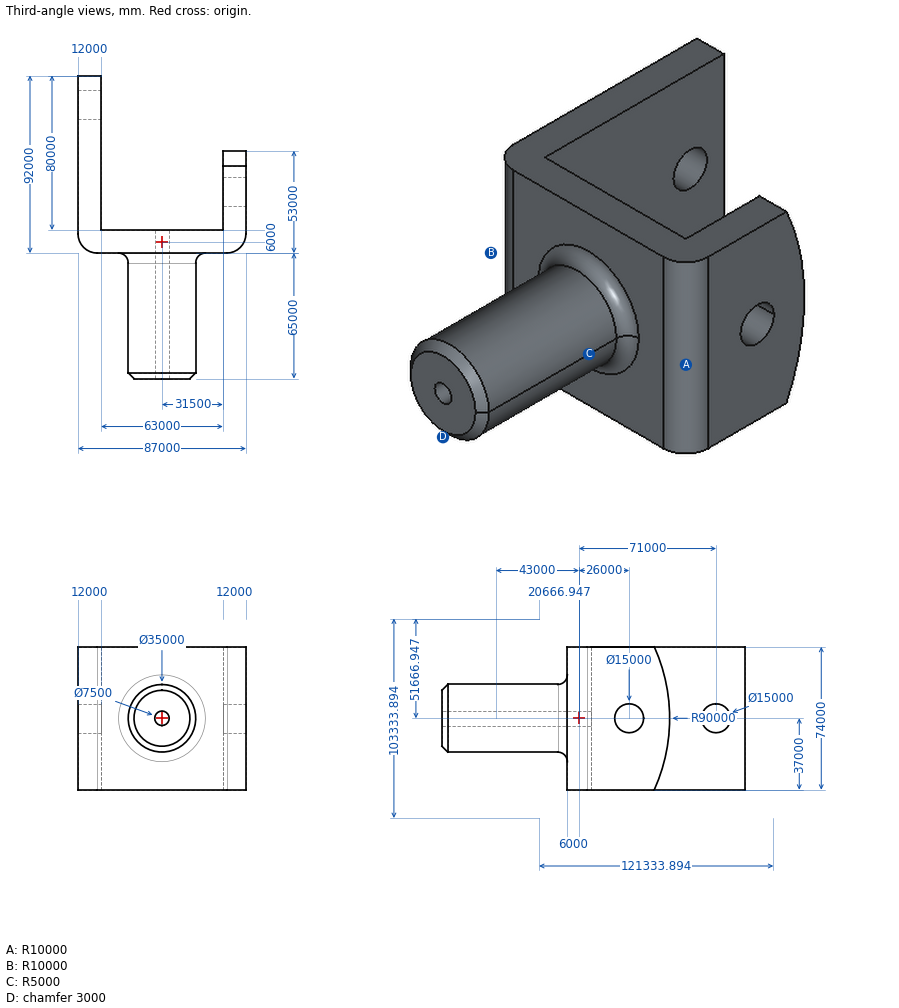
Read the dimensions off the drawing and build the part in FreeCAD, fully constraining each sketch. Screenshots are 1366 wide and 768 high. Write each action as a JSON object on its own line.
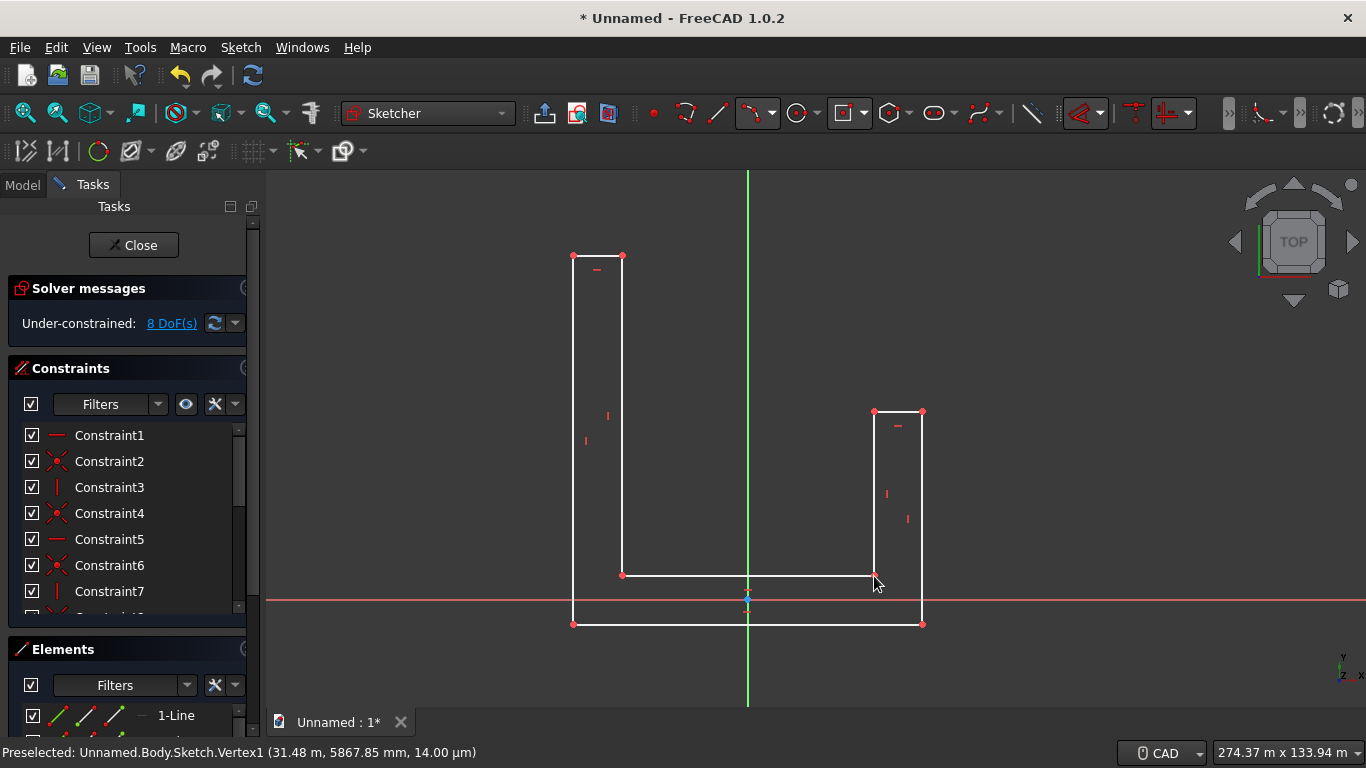
{"action": "left_click", "coordinate": [1080, 114]}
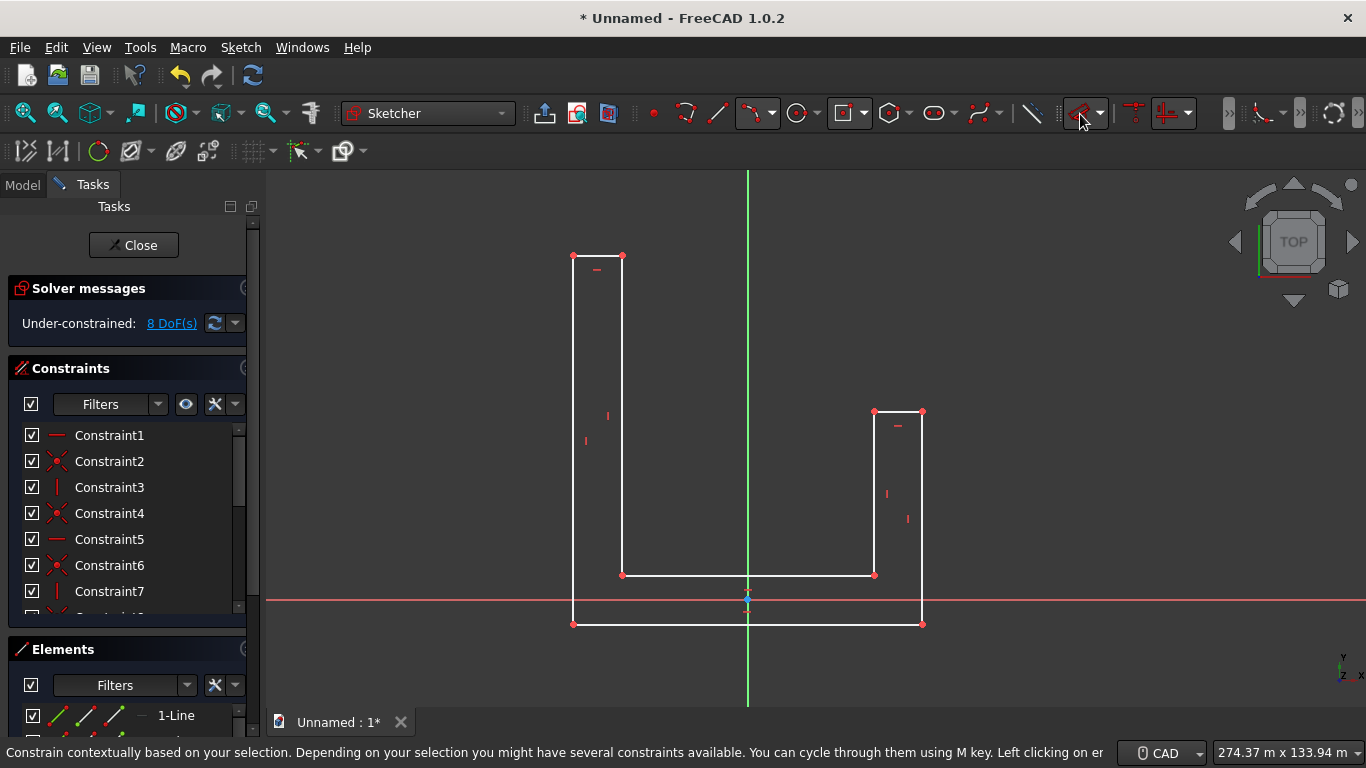
{"action": "left_click", "coordinate": [798, 576]}
{"action": "left_click", "coordinate": [690, 542]}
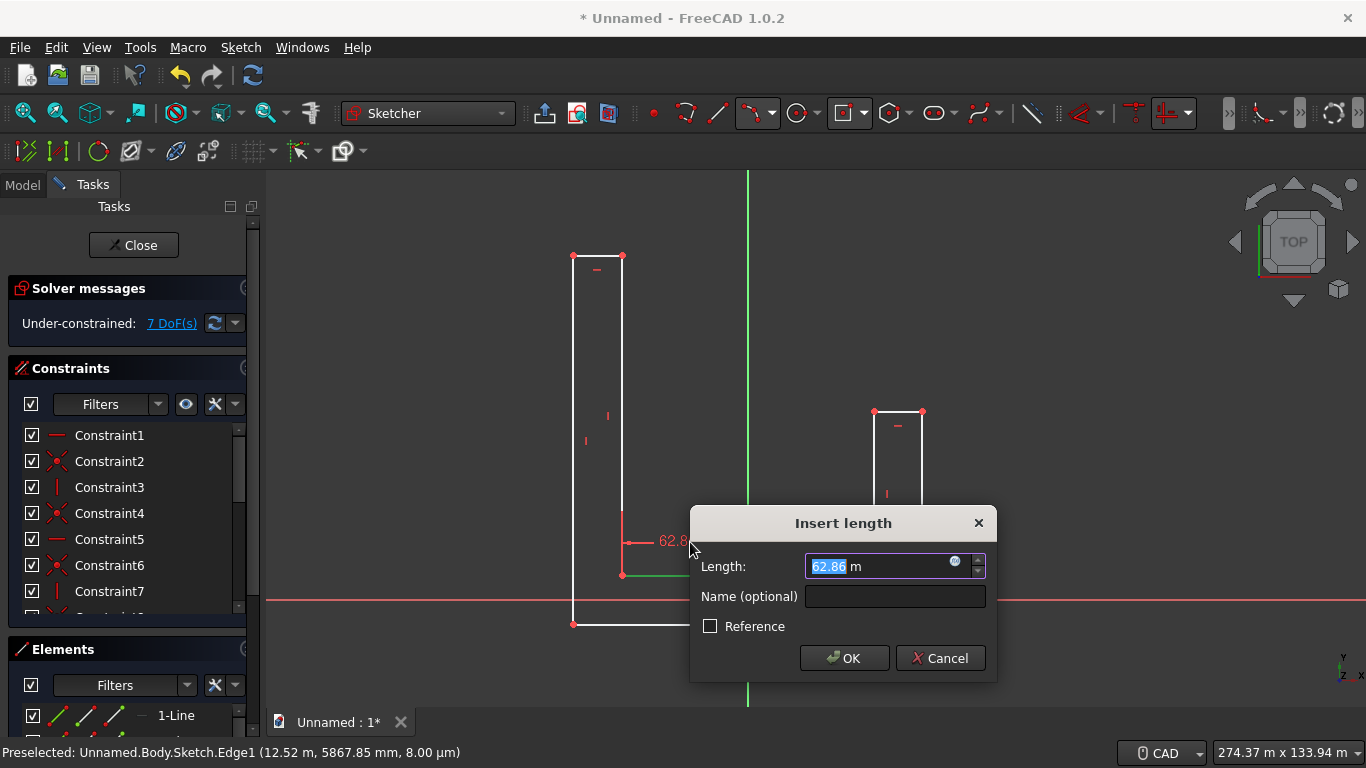
{"action": "key", "text": "ctrl+a"}
{"action": "type", "text": "63000 mm"}
{"action": "key", "text": "Return"}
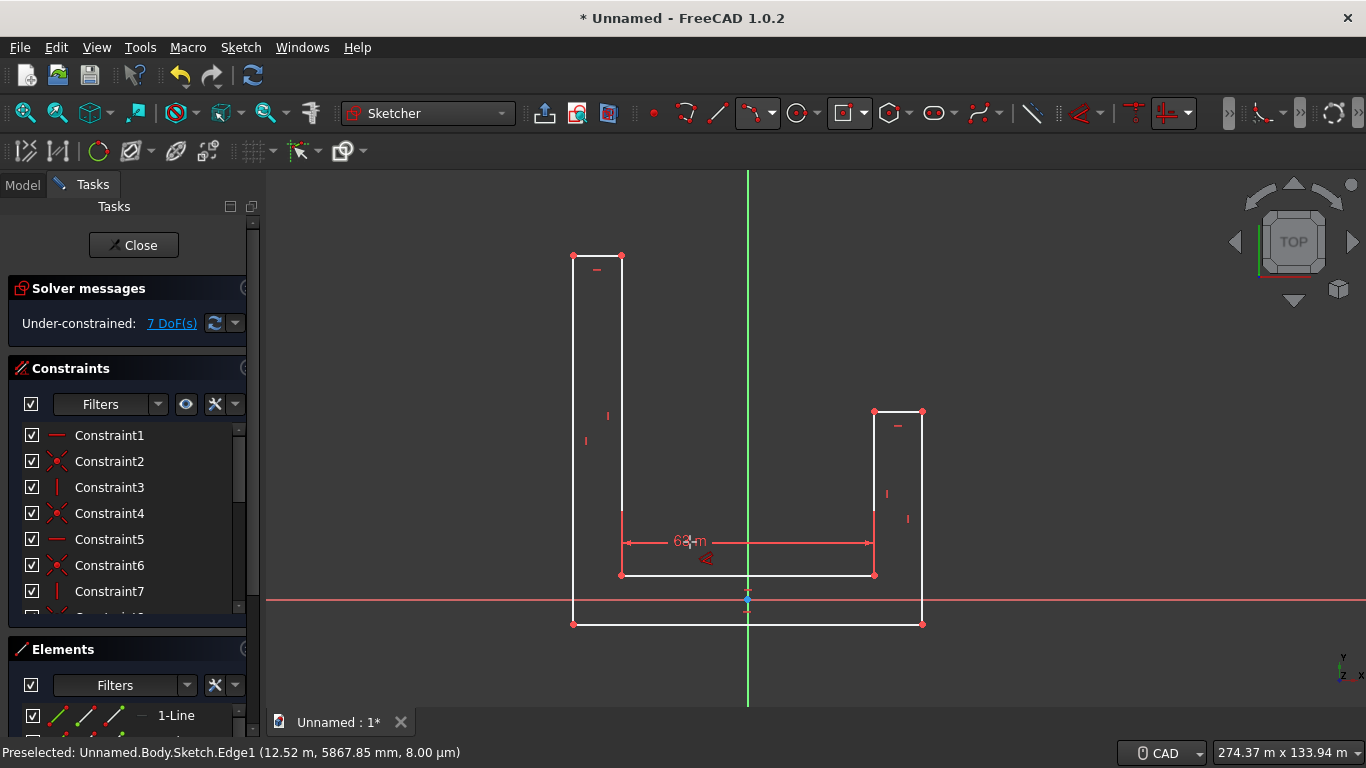
{"action": "left_click", "coordinate": [622, 480]}
{"action": "left_click", "coordinate": [588, 416]}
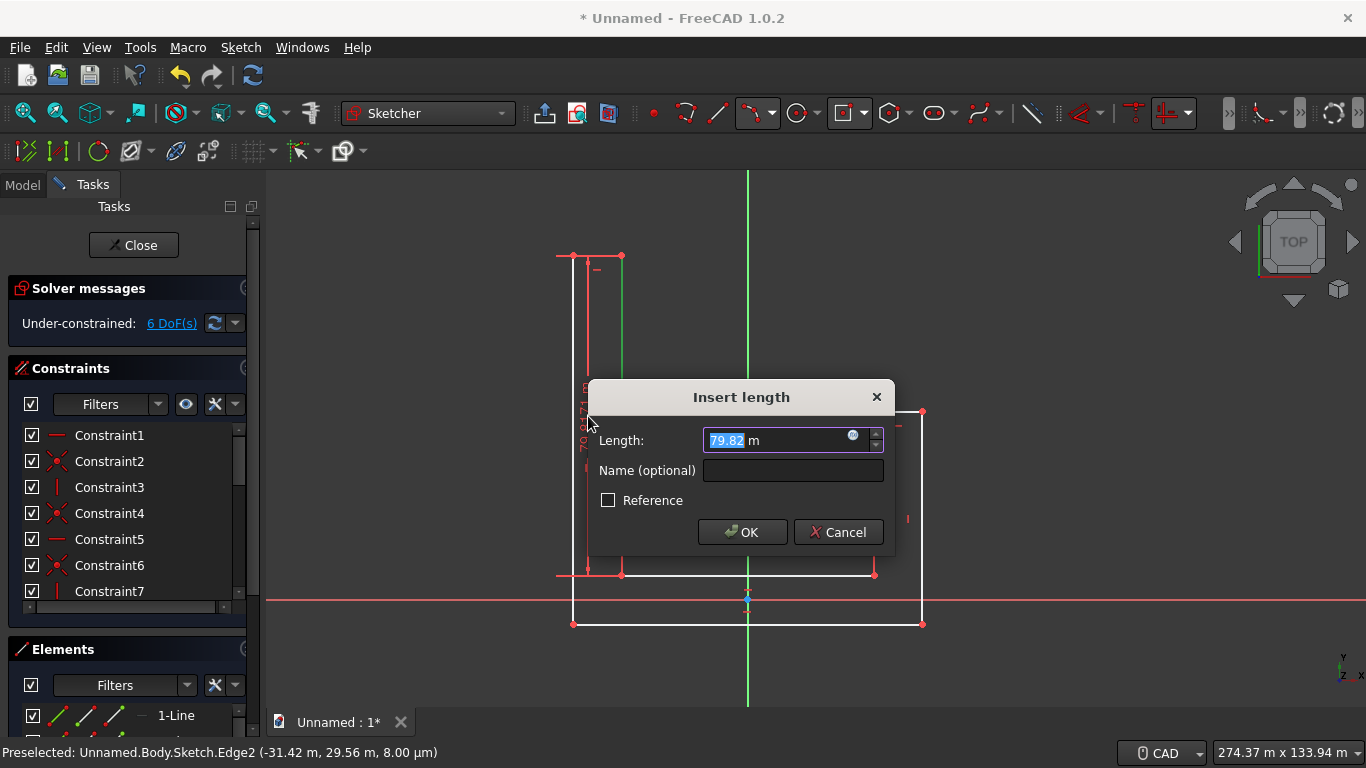
{"action": "key", "text": "ctrl+a"}
{"action": "type", "text": "80000 mm"}
{"action": "key", "text": "Return"}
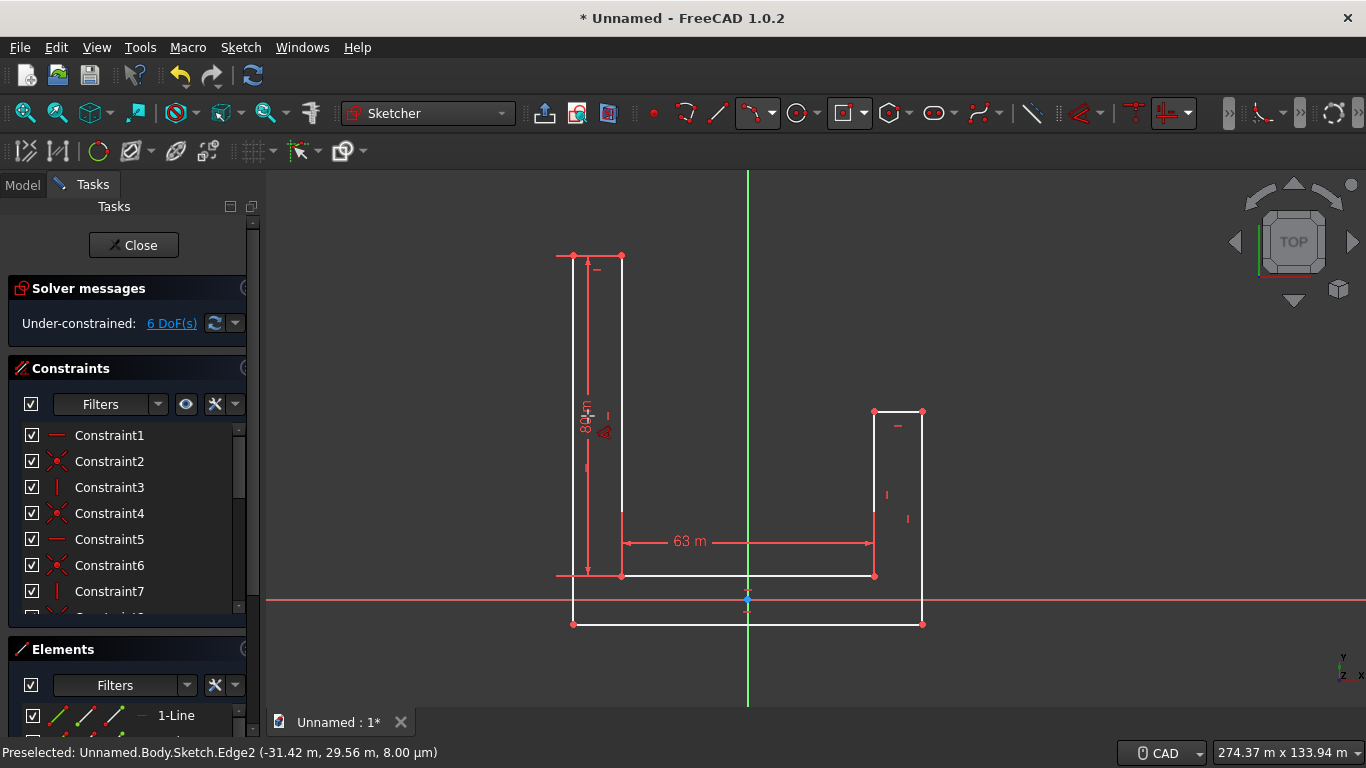
{"action": "left_click", "coordinate": [607, 256]}
{"action": "left_click", "coordinate": [597, 222]}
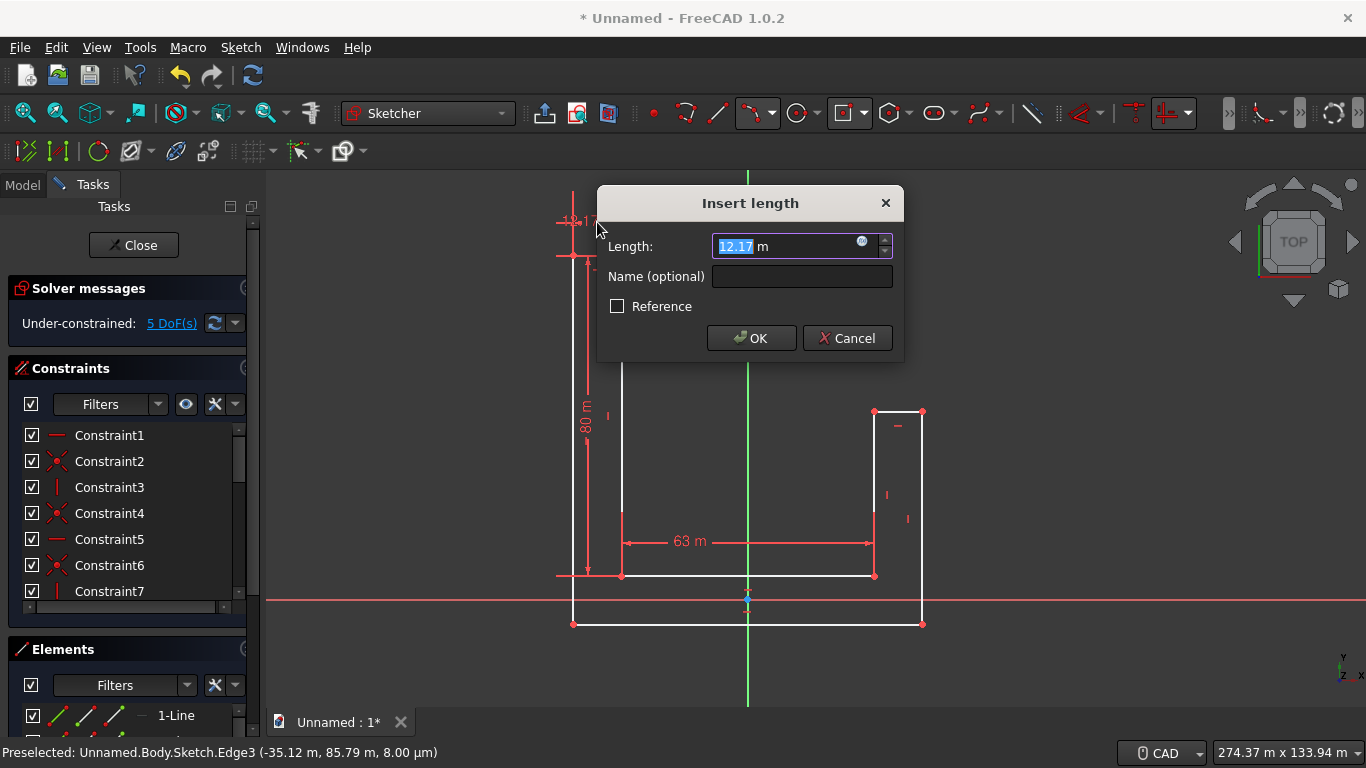
{"action": "key", "text": "ctrl+a"}
{"action": "type", "text": "12000 mm"}
{"action": "key", "text": "Return"}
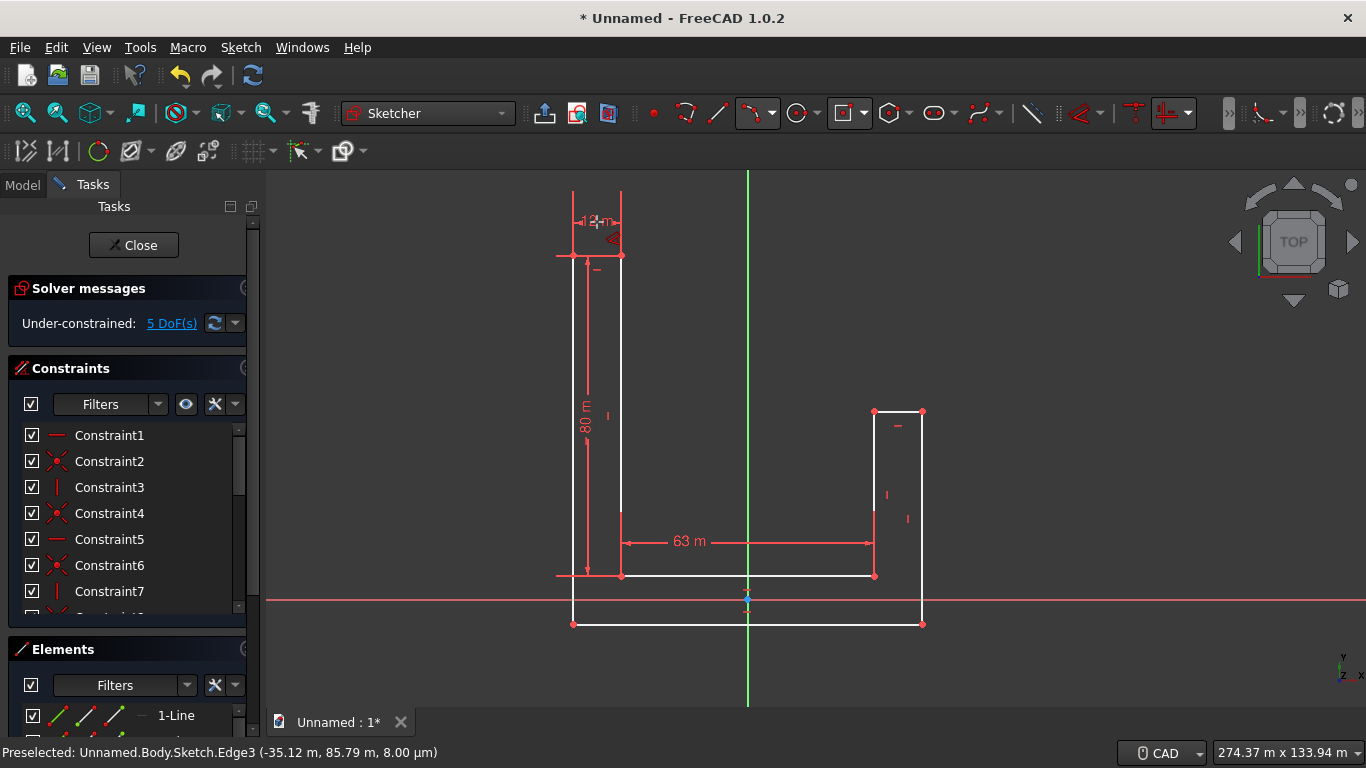
{"action": "left_click", "coordinate": [573, 366]}
{"action": "left_click", "coordinate": [539, 440]}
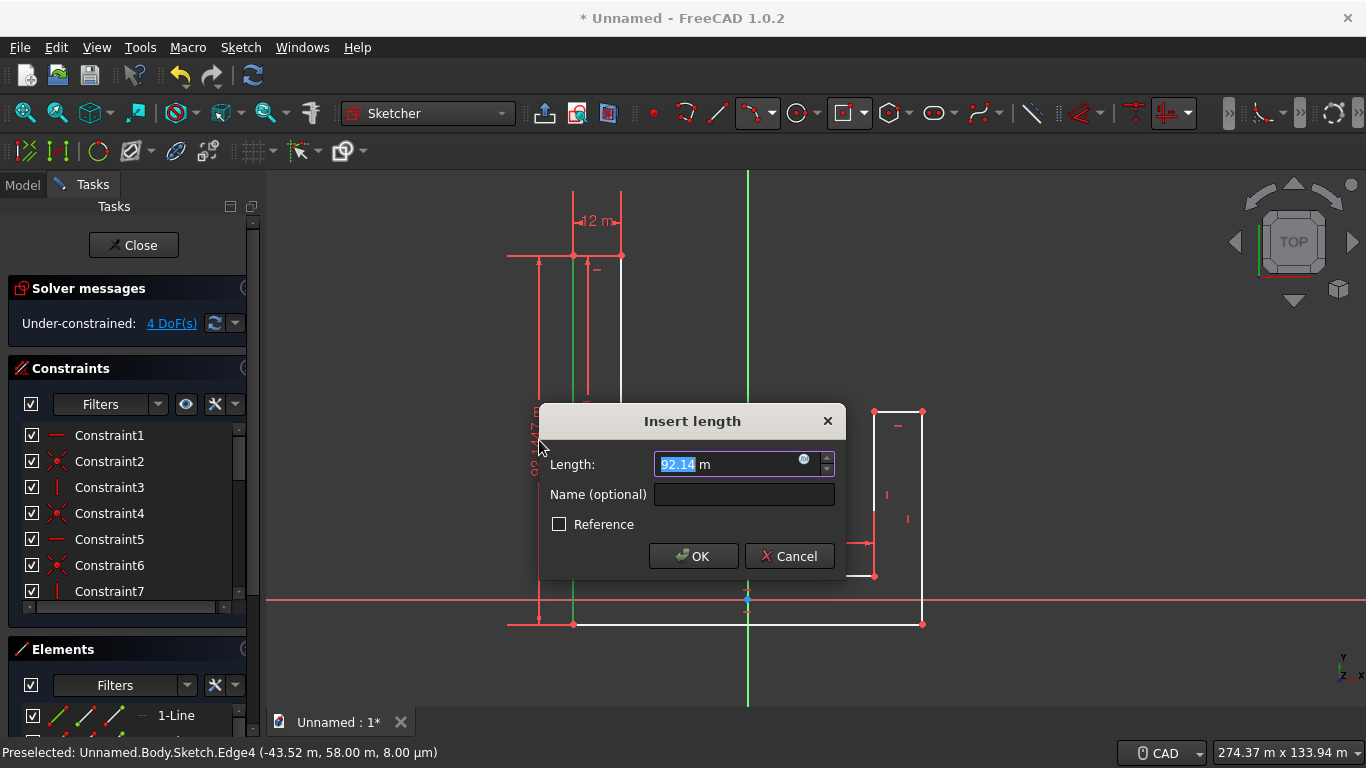
{"action": "key", "text": "ctrl+a"}
{"action": "type", "text": "92000 mm"}
{"action": "key", "text": "Return"}